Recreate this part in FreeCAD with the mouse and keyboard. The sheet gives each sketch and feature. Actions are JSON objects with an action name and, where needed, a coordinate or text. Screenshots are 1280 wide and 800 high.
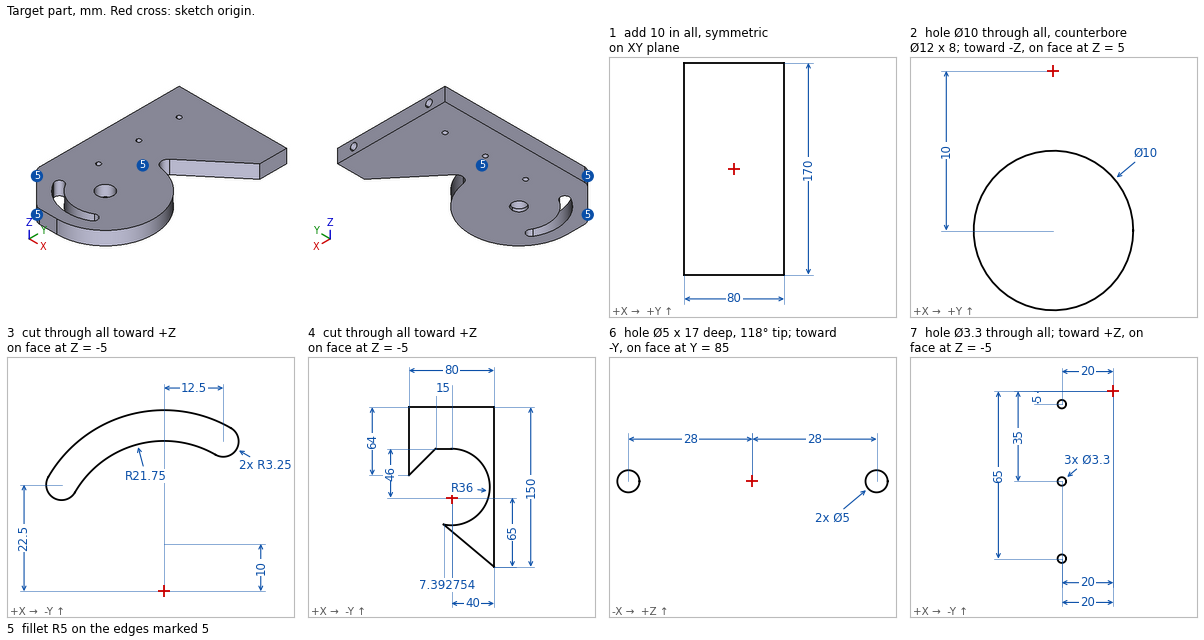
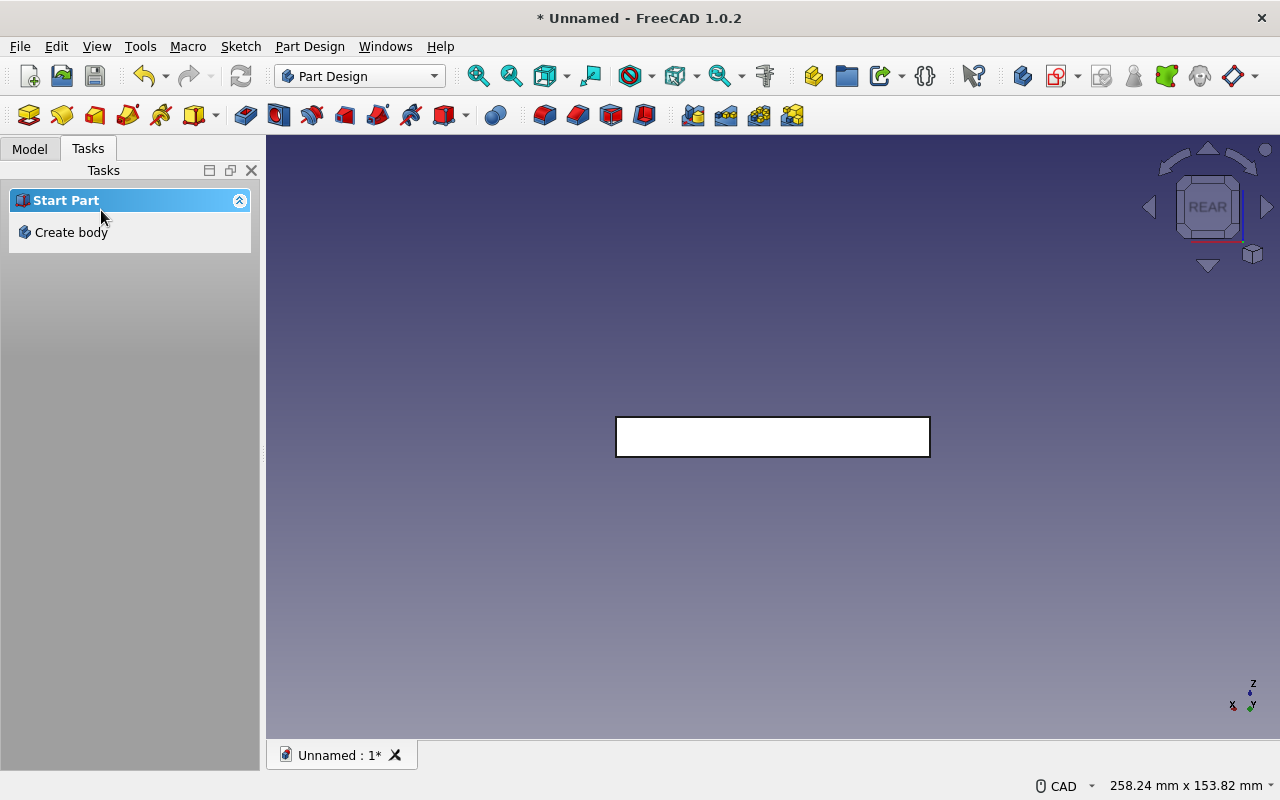
{"action": "key", "text": "v f"}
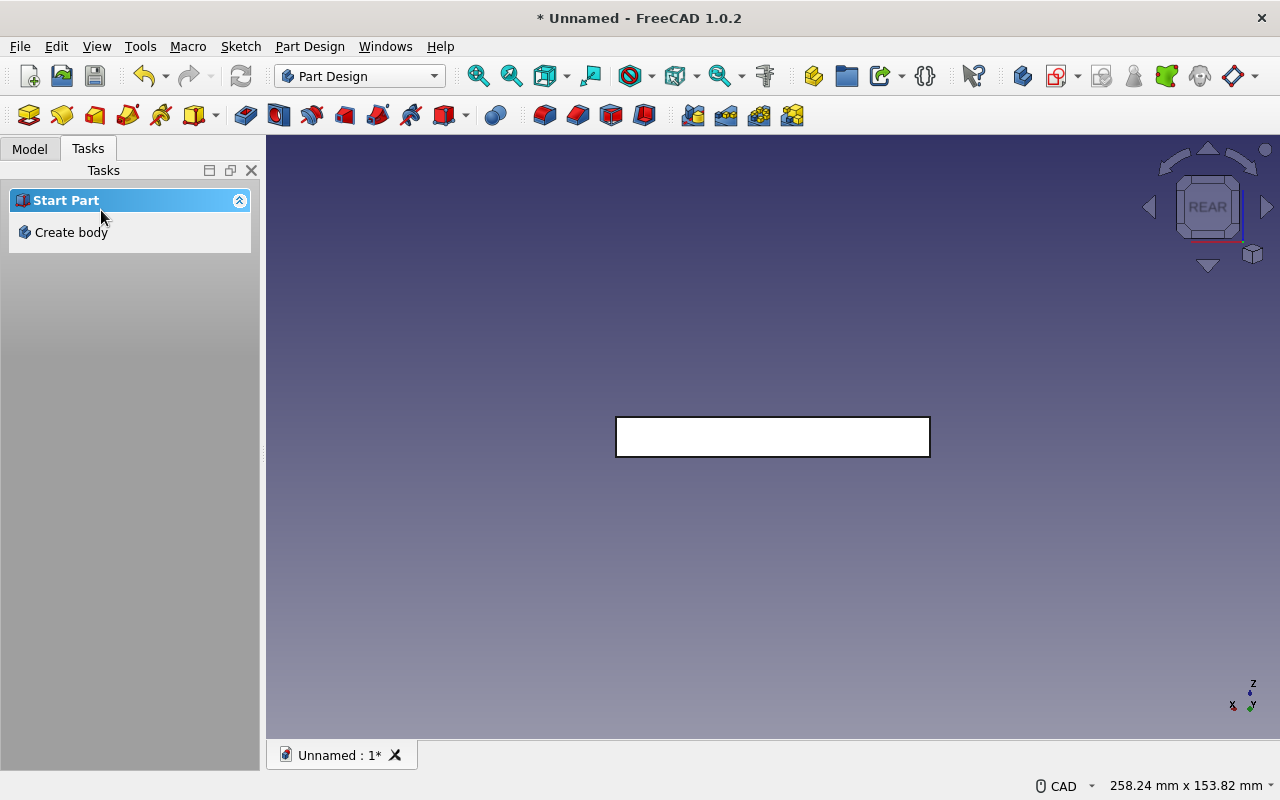
{"action": "left_click", "coordinate": [638, 436]}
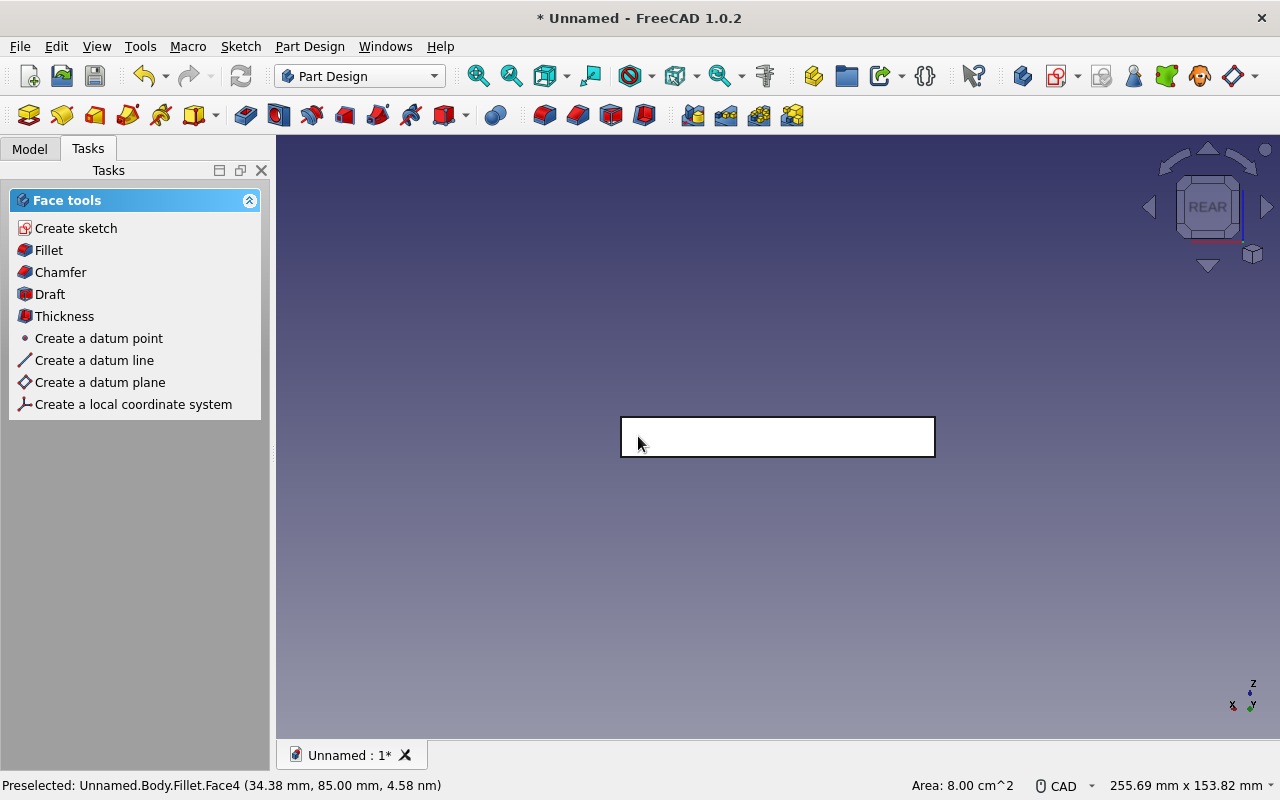
{"action": "left_click", "coordinate": [1056, 76]}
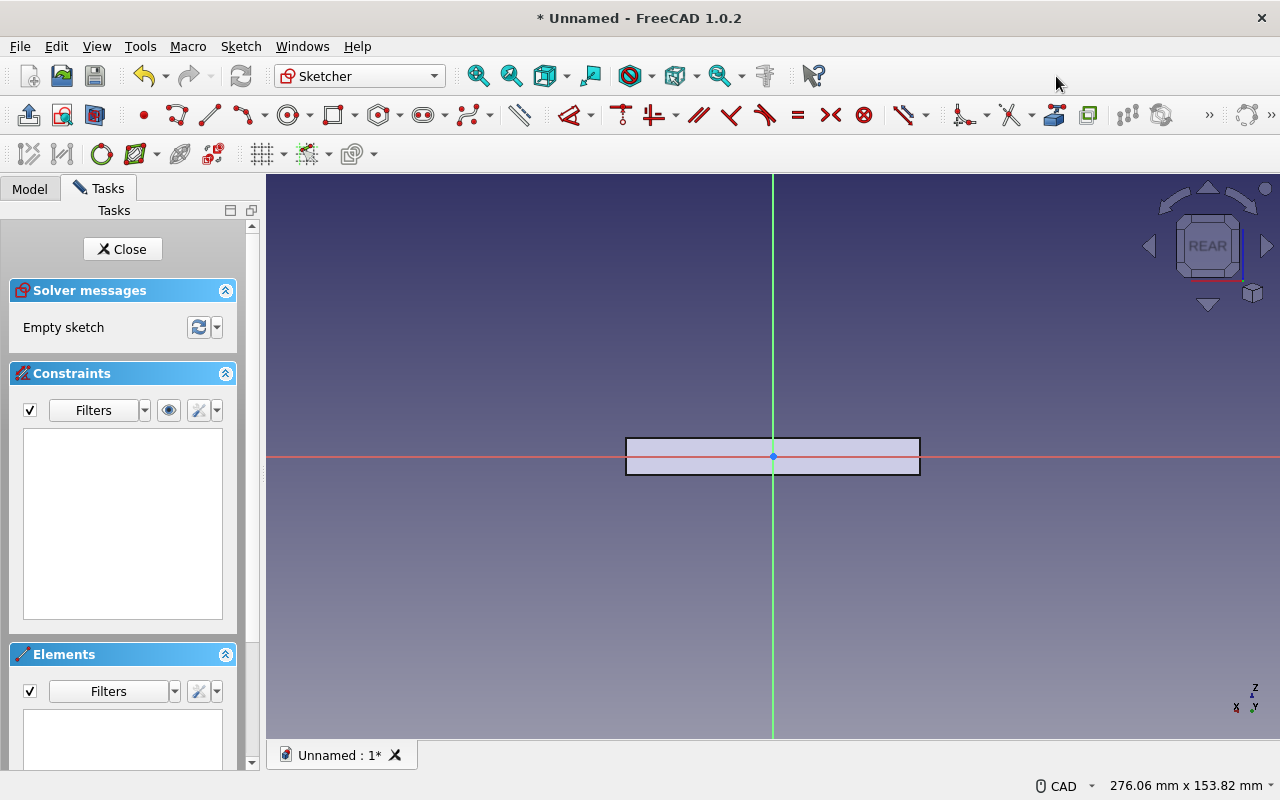
{"action": "scroll", "coordinate": [813, 456], "scroll_direction": "up", "scroll_amount": 5}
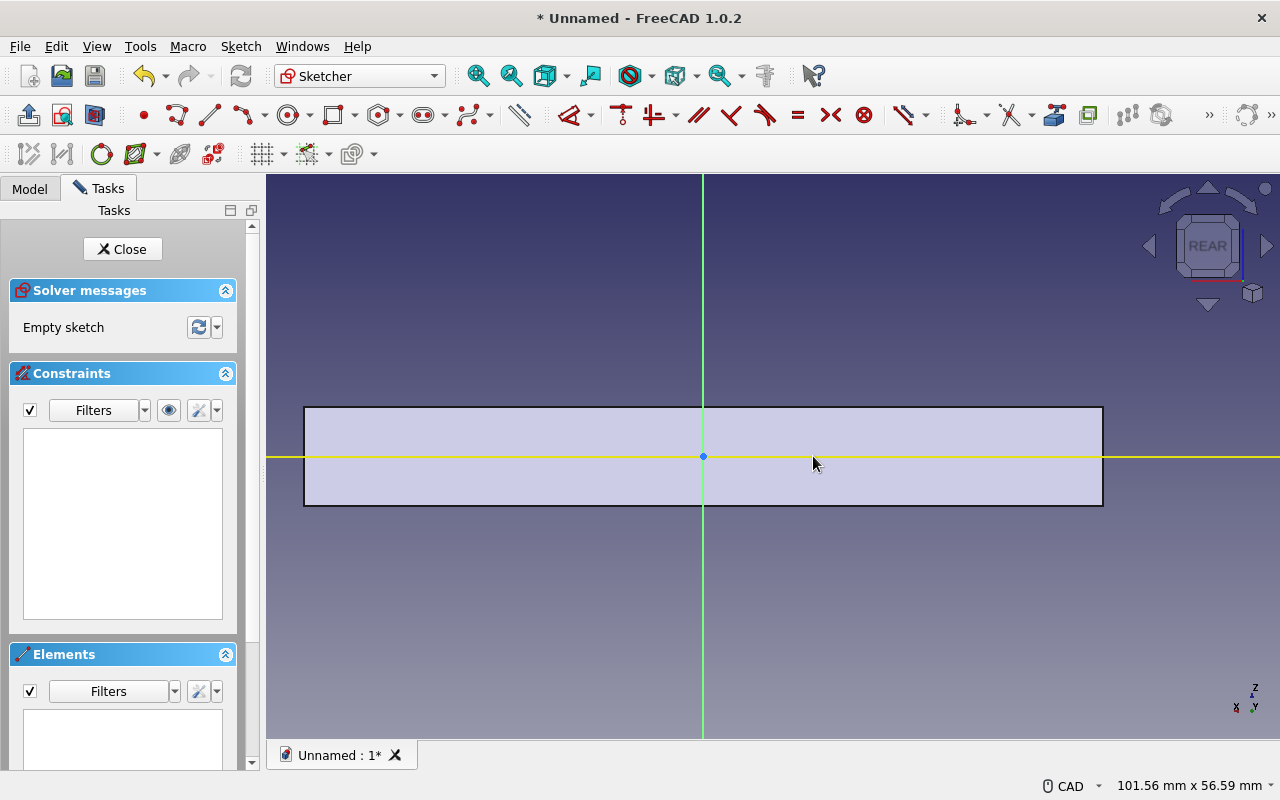
{"action": "key", "text": "g c"}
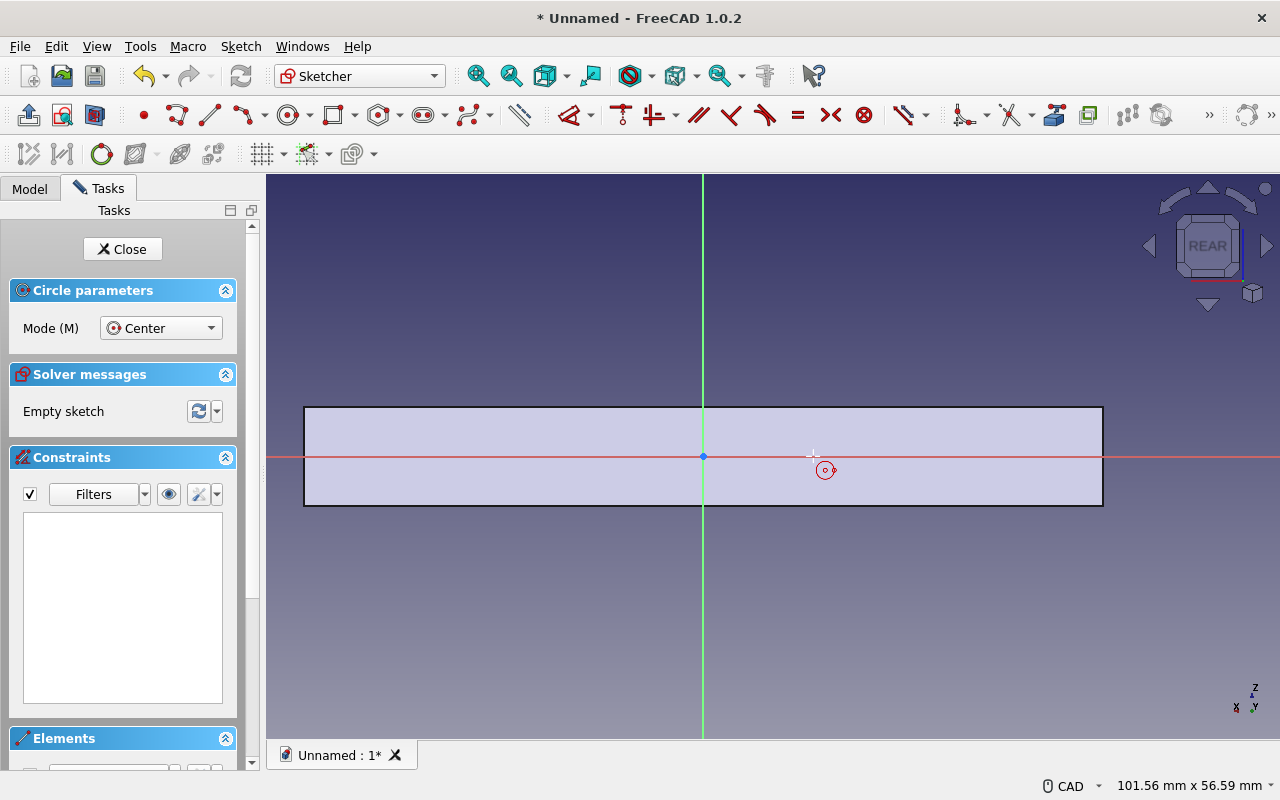
{"action": "left_click", "coordinate": [983, 456]}
{"action": "left_click", "coordinate": [1001, 439]}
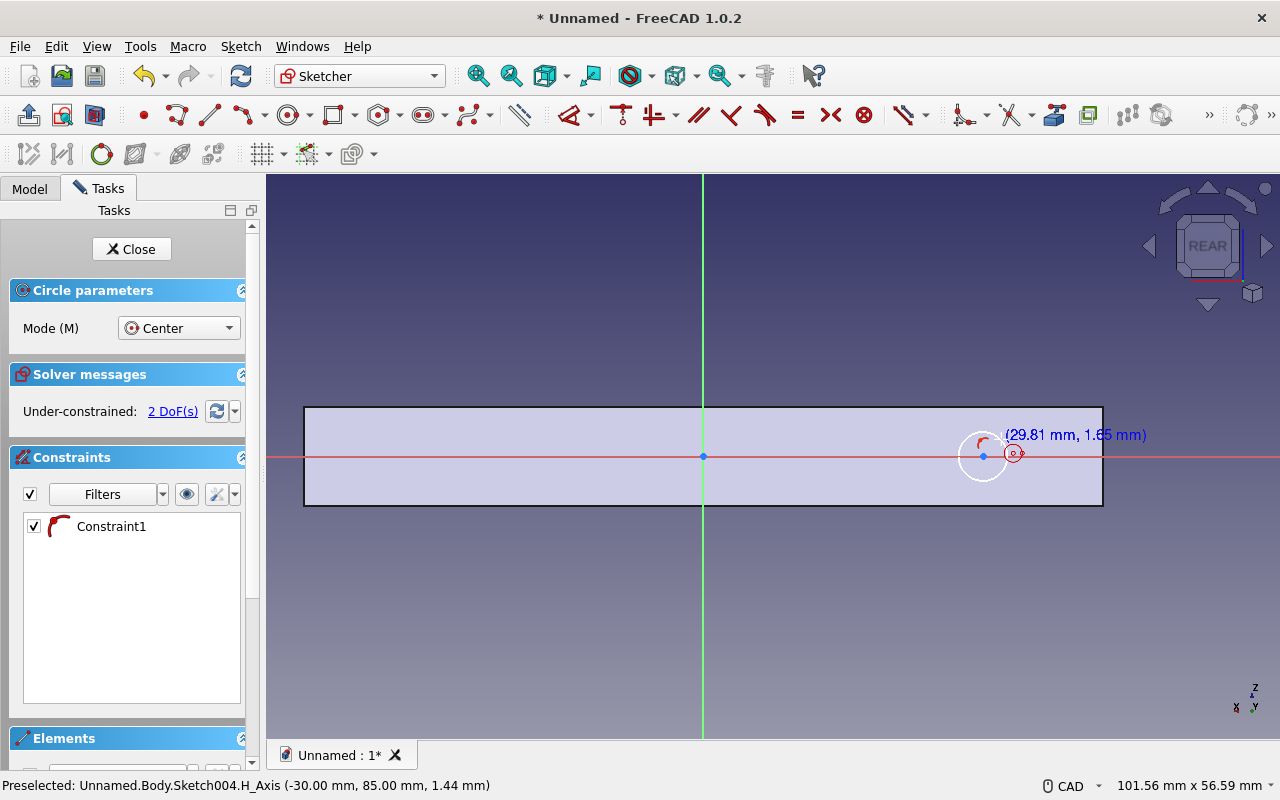
{"action": "left_click", "coordinate": [424, 456]}
{"action": "left_click", "coordinate": [441, 439]}
{"action": "key", "text": "Escape"}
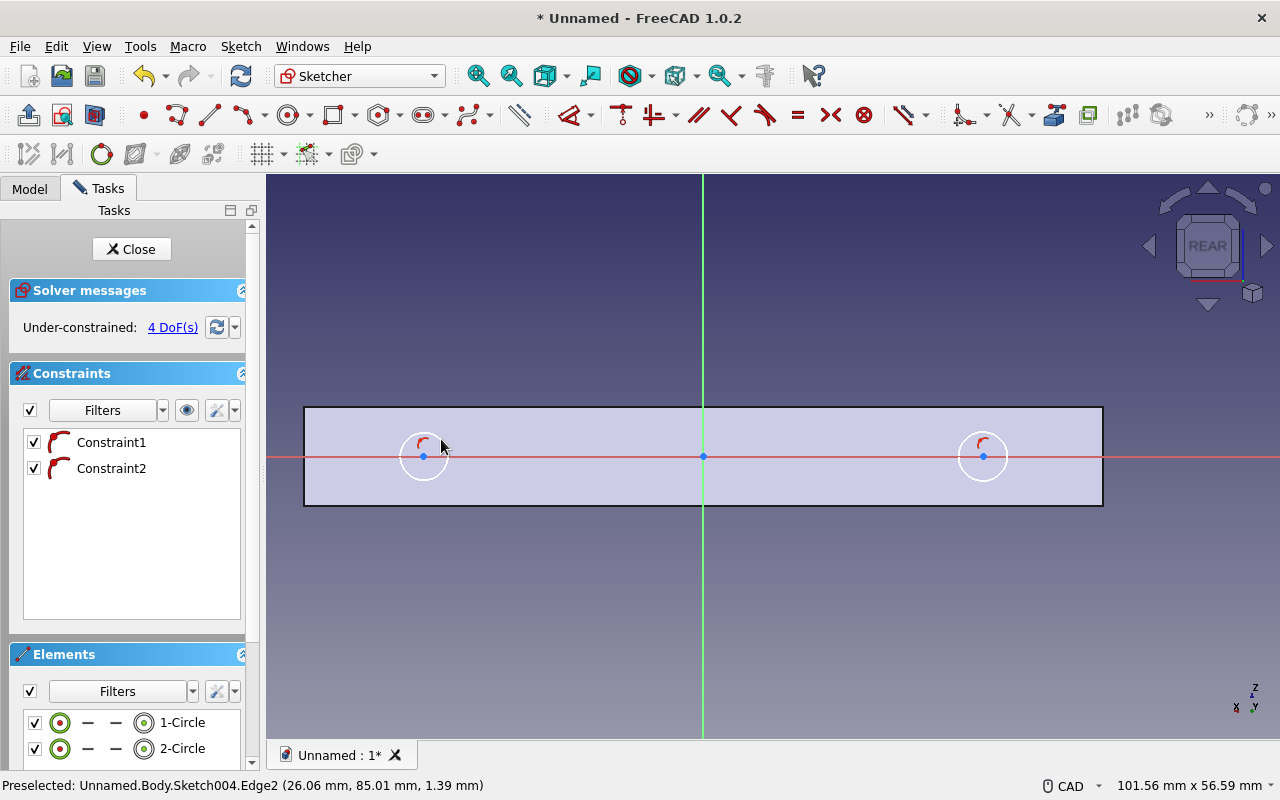
{"action": "left_click", "coordinate": [1000, 439]}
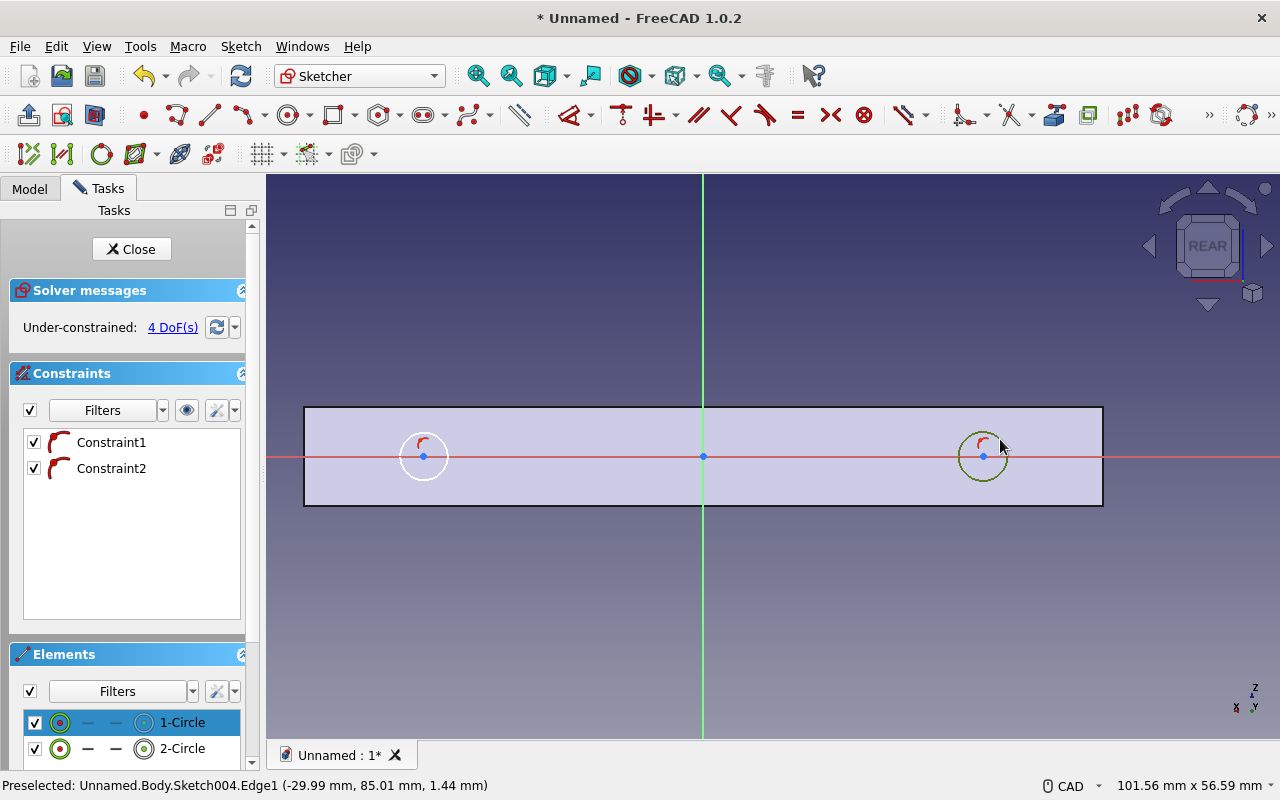
{"action": "left_click", "coordinate": [441, 440]}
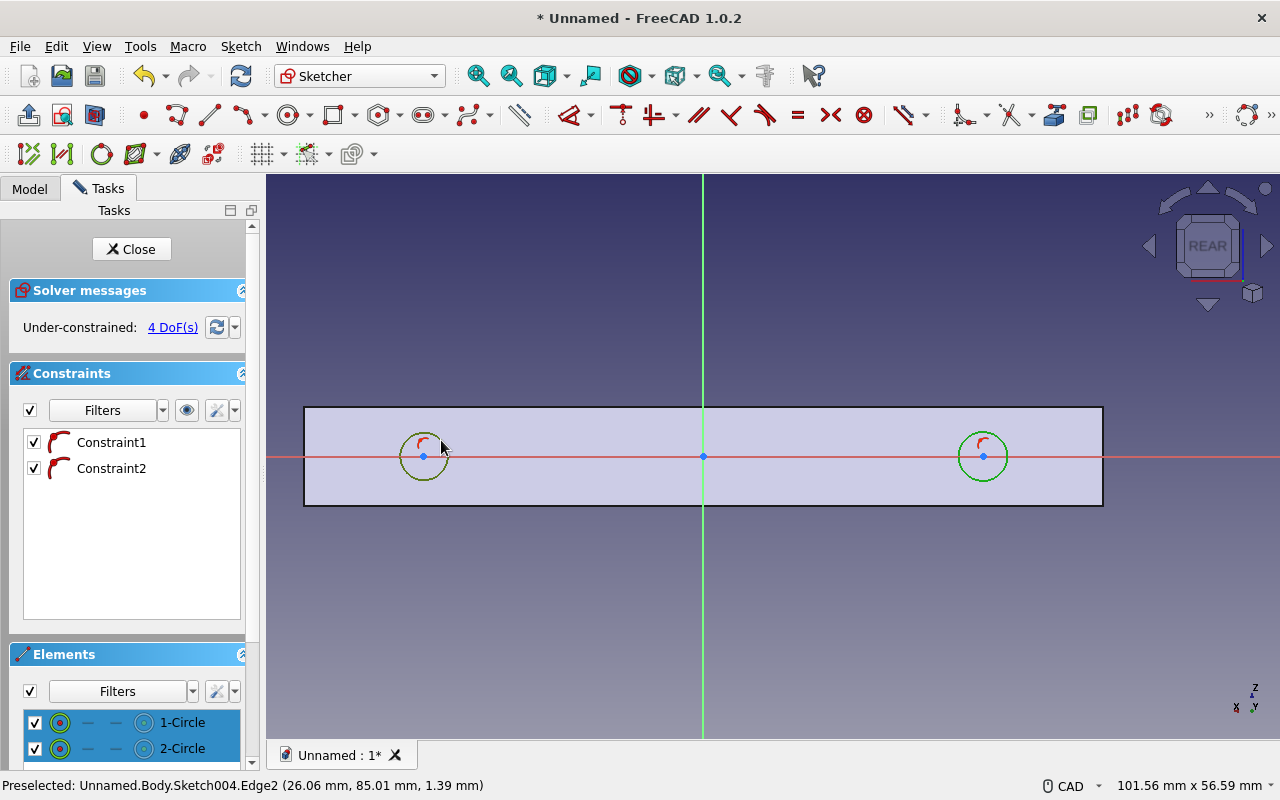
{"action": "key", "text": "e"}